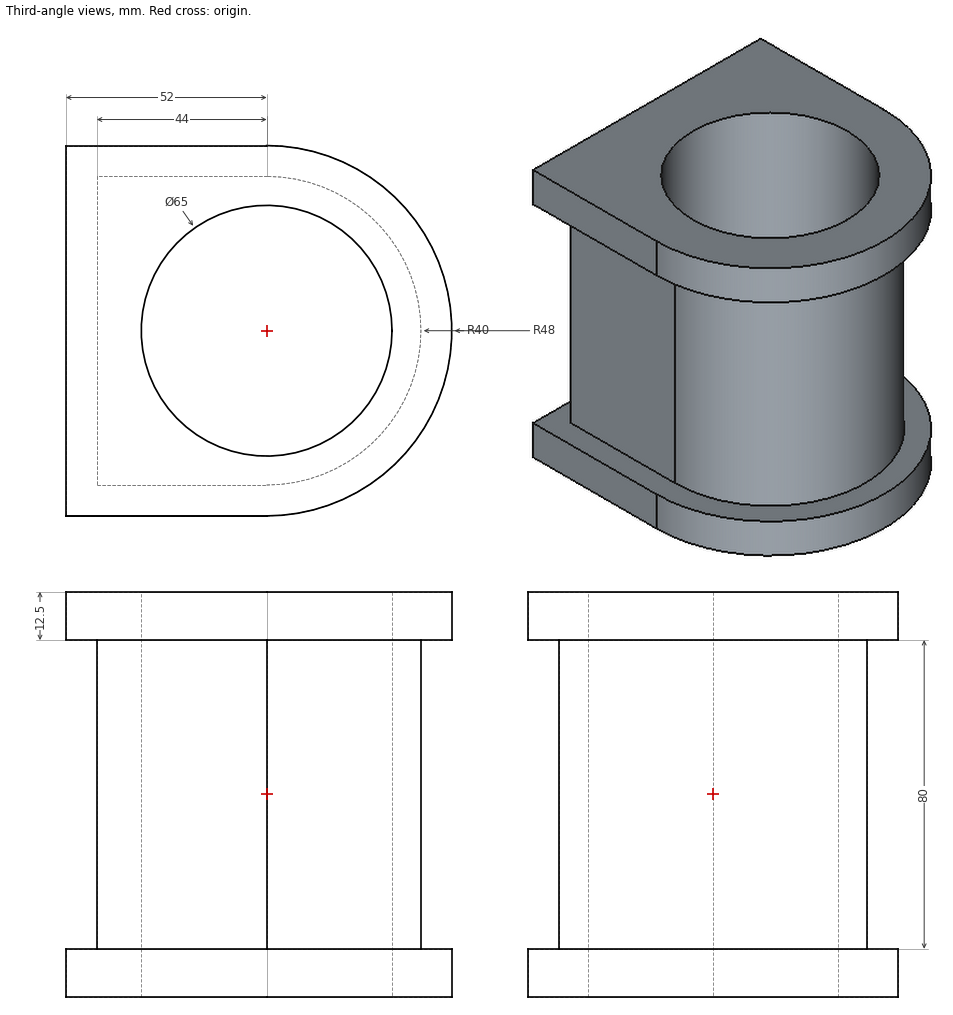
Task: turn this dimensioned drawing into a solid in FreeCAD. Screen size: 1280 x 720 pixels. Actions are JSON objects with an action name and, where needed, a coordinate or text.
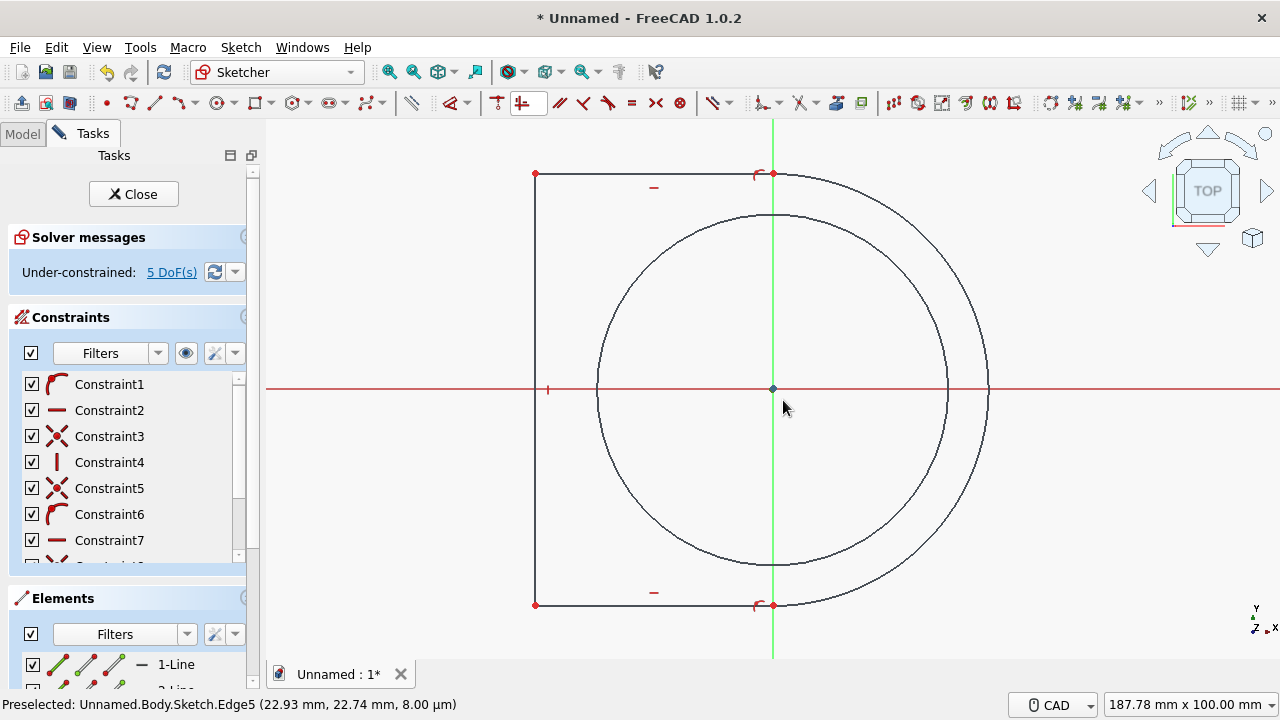
{"action": "left_click", "coordinate": [498, 104]}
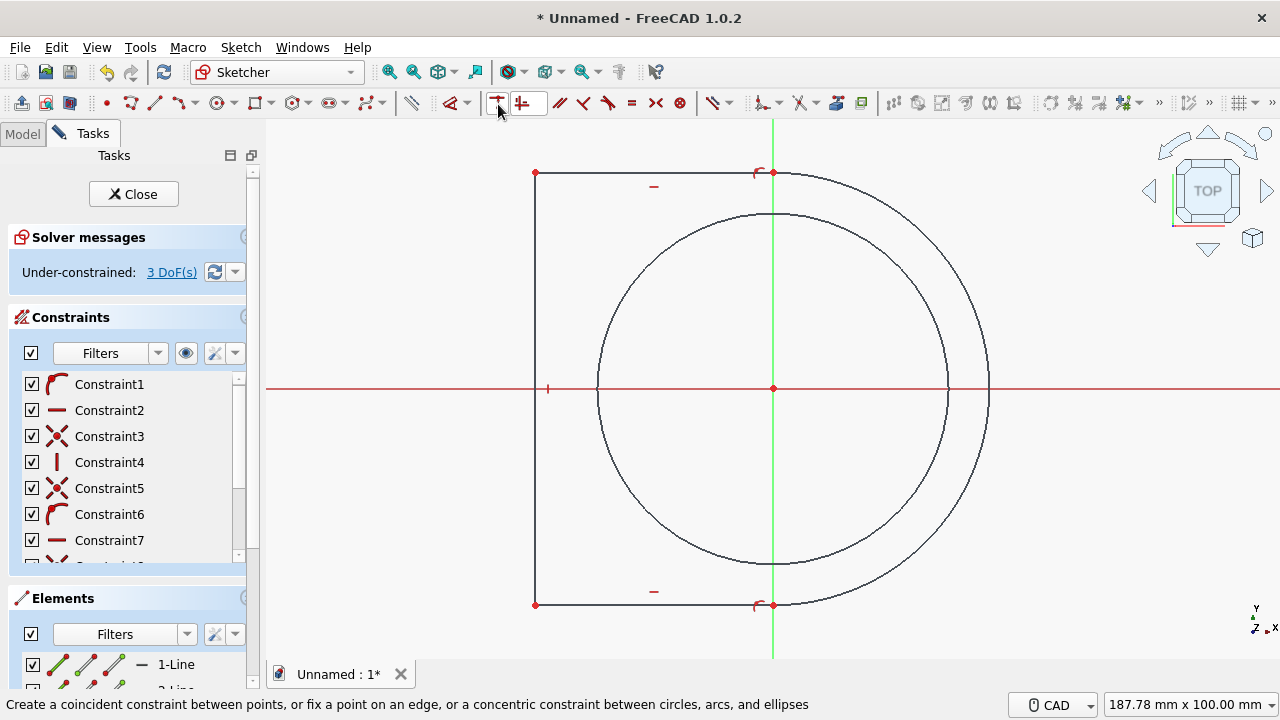
{"action": "left_click", "coordinate": [948, 516]}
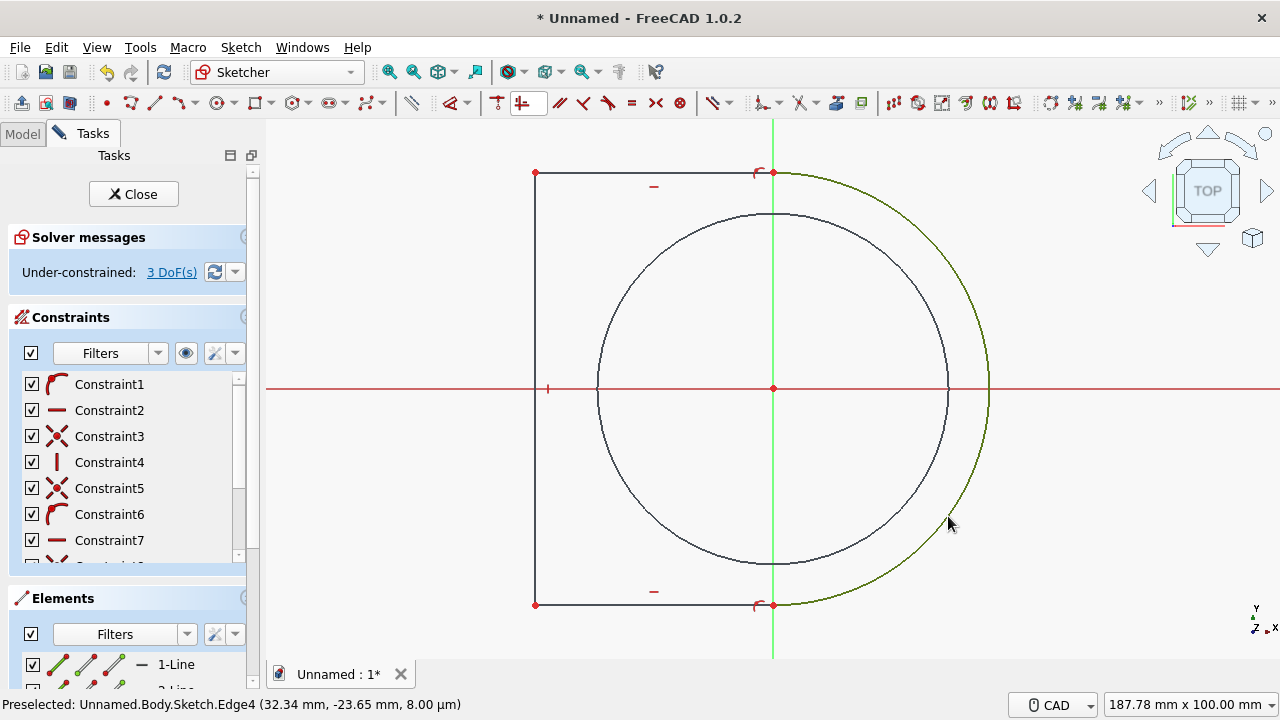
{"action": "key", "text": "k r"}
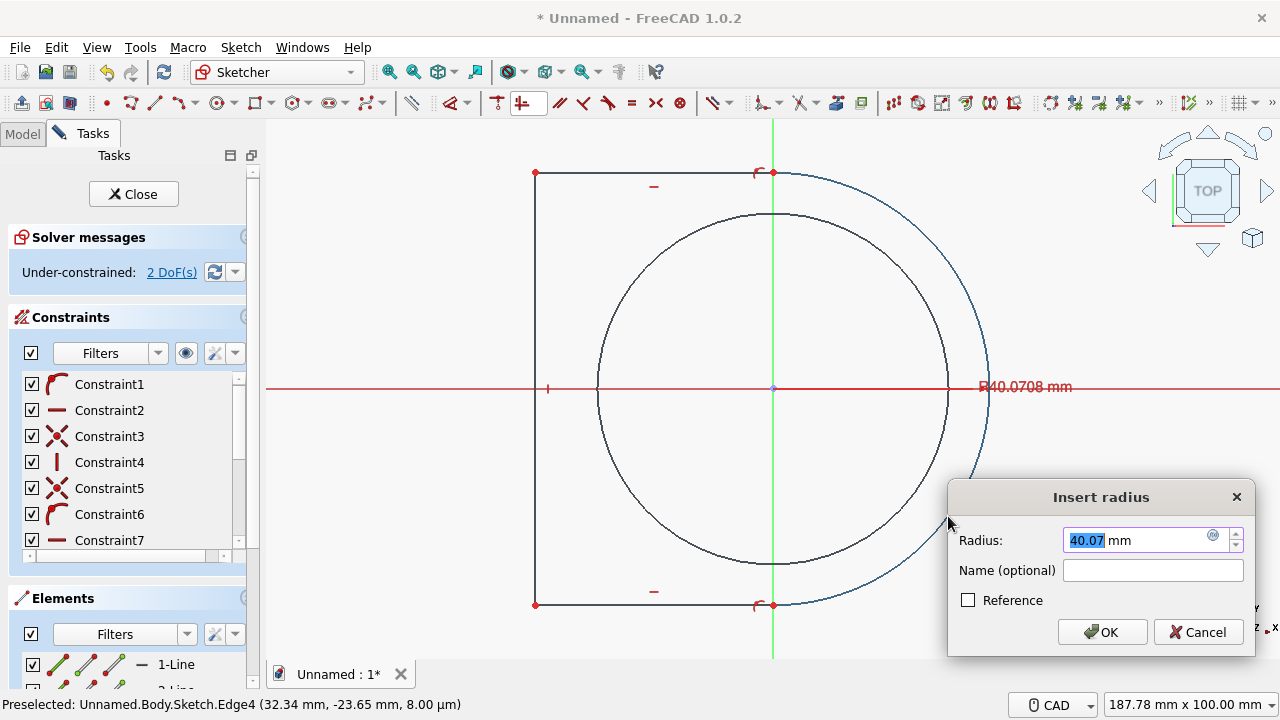
{"action": "type", "text": "40"}
{"action": "key", "text": "Return"}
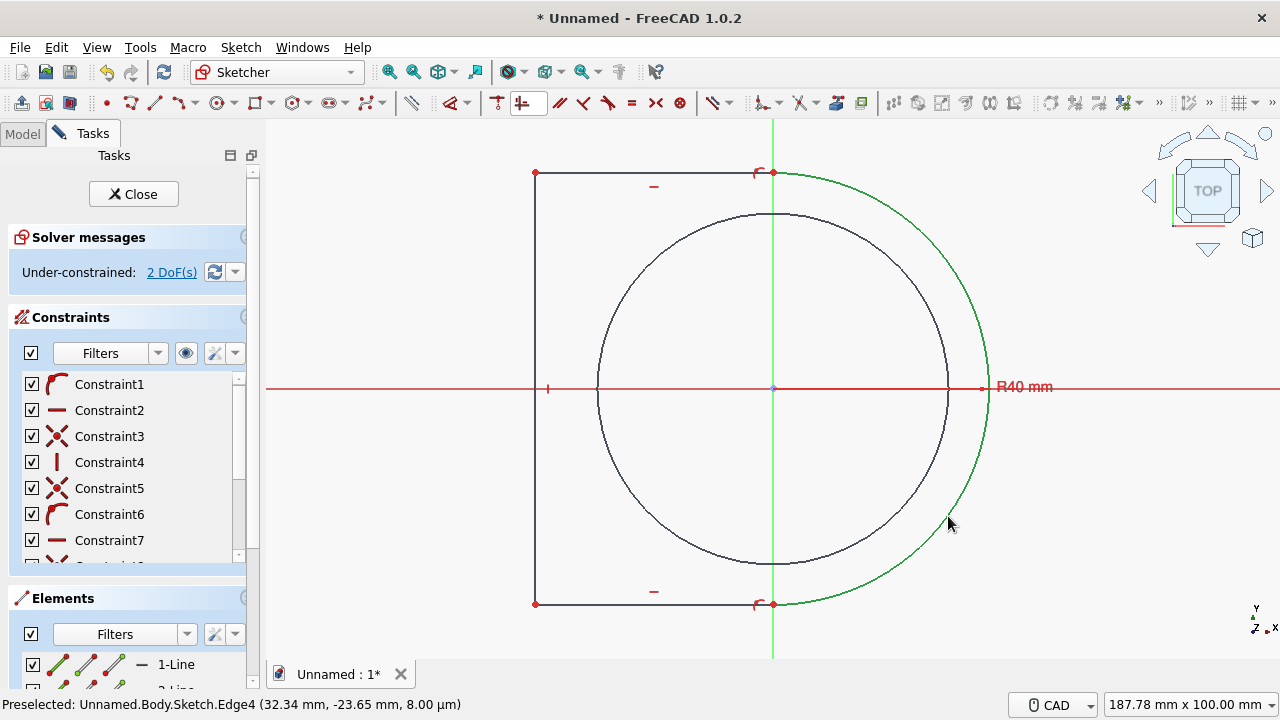
{"action": "left_click", "coordinate": [897, 264]}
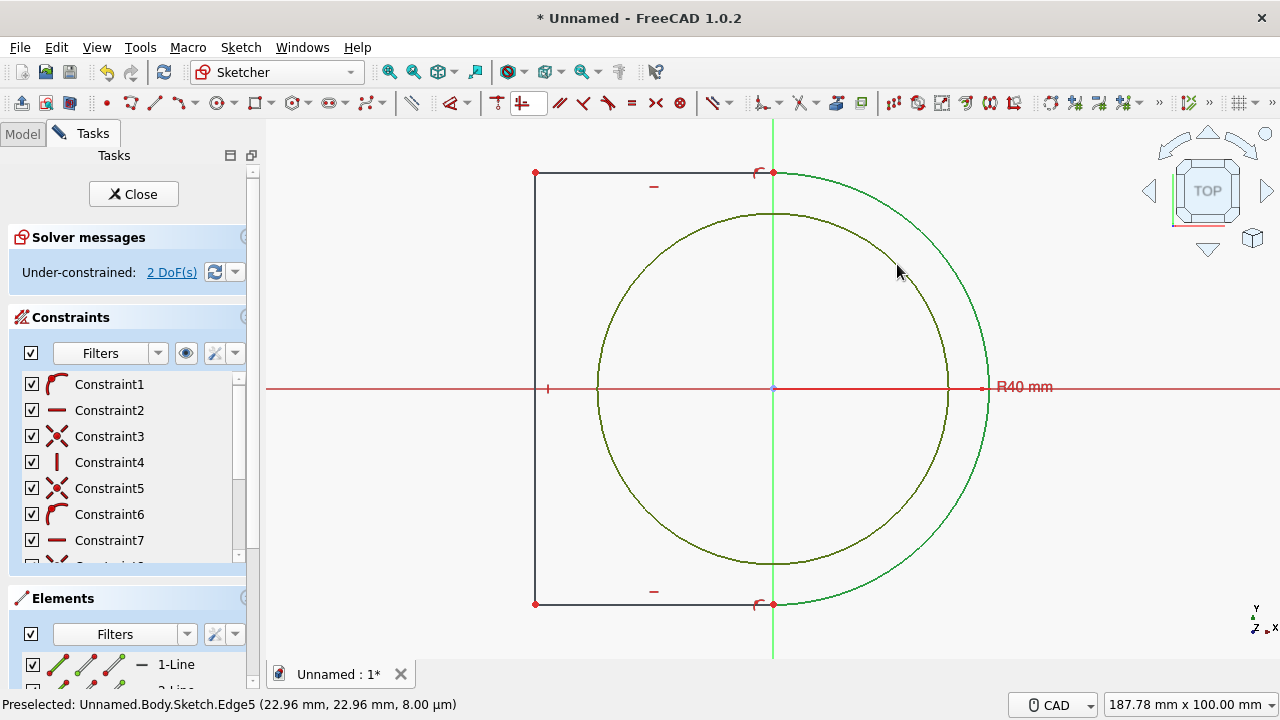
{"action": "key", "text": "k o"}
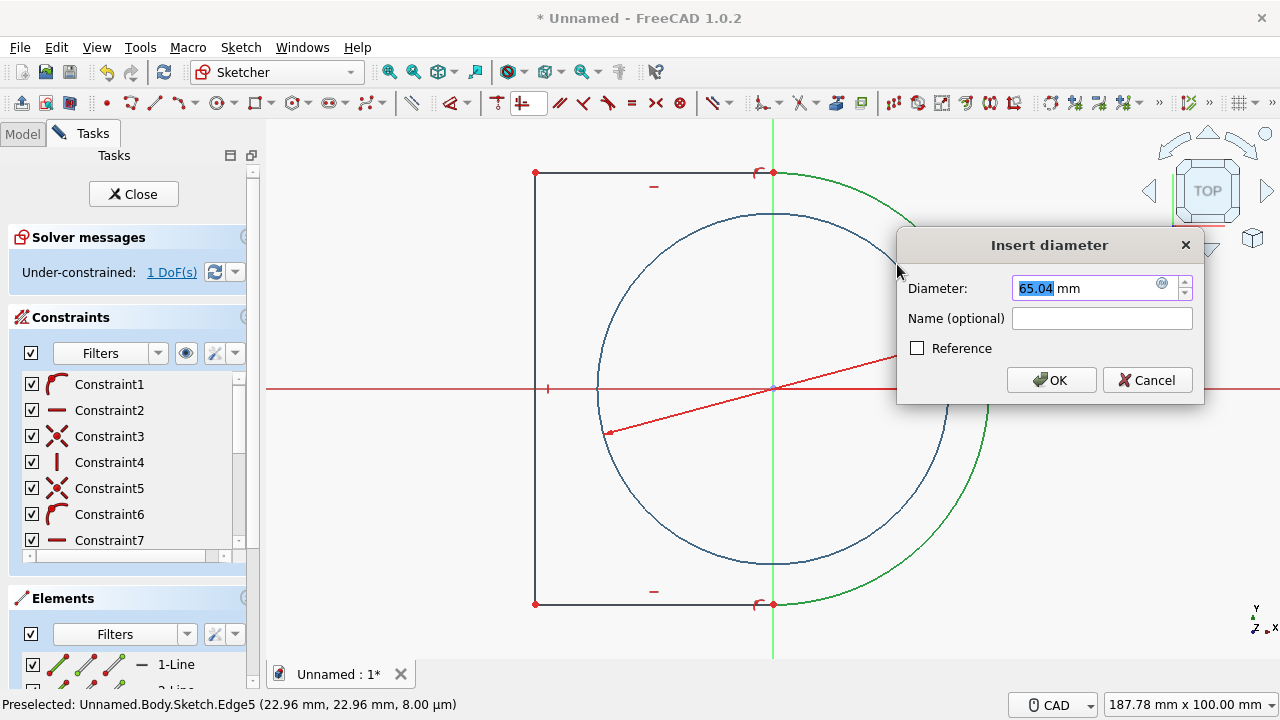
{"action": "type", "text": "65"}
{"action": "key", "text": "Return"}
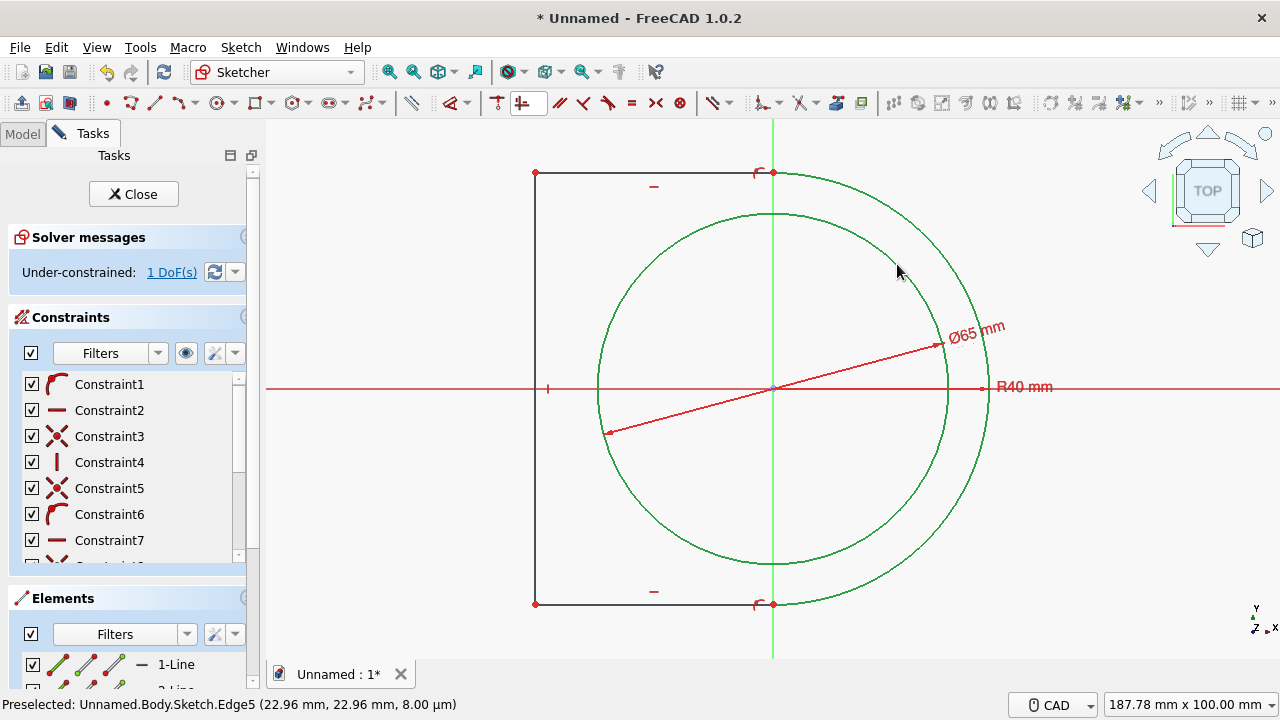
{"action": "left_click", "coordinate": [702, 173]}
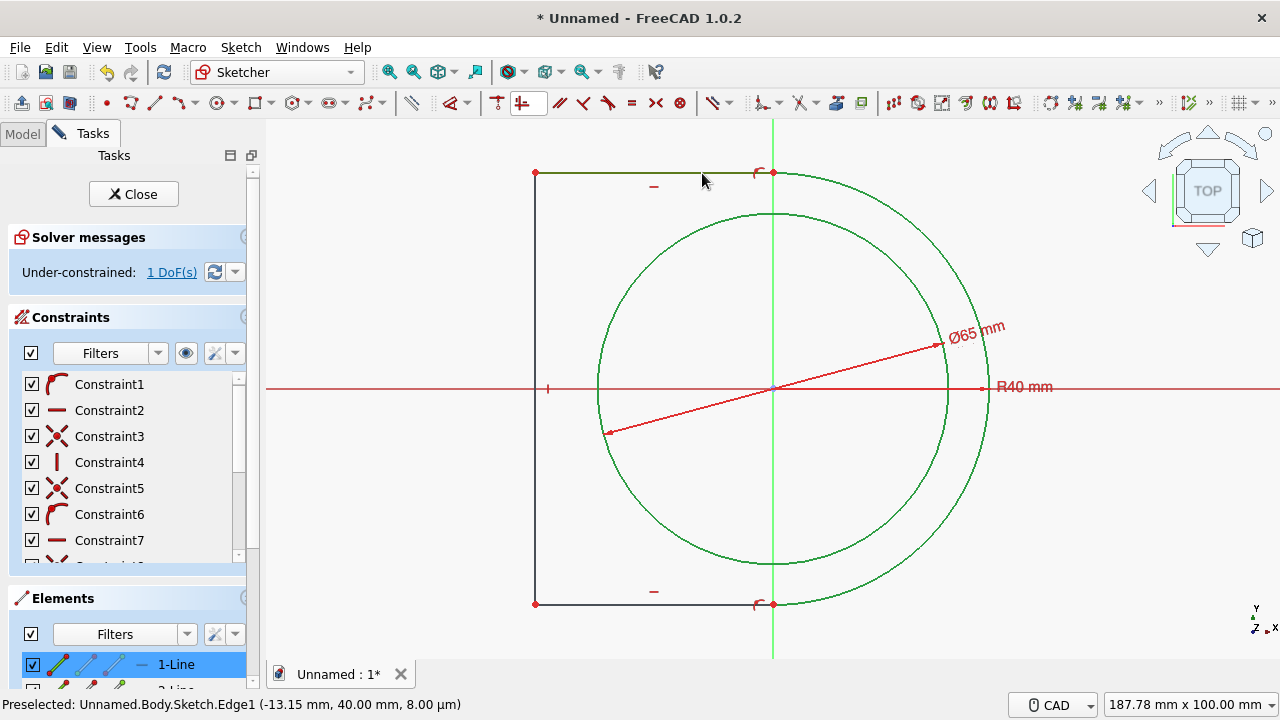
{"action": "key", "text": "l"}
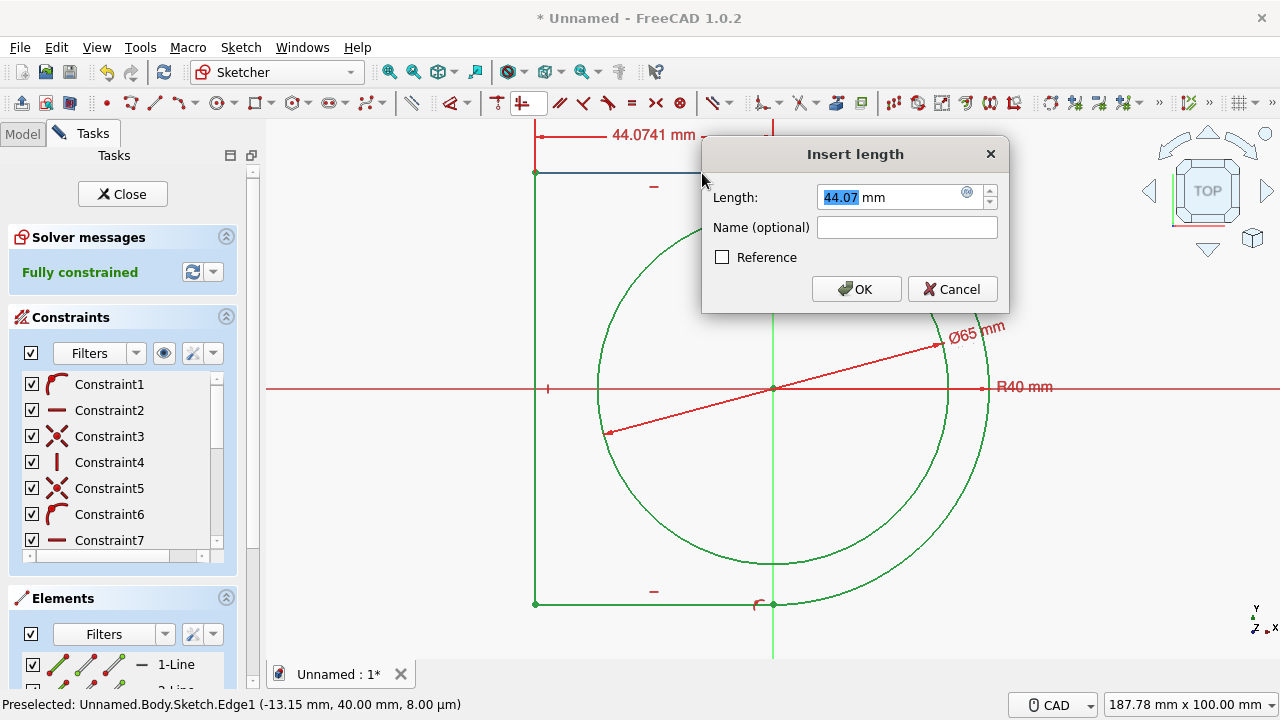
{"action": "type", "text": "44"}
{"action": "key", "text": "Return"}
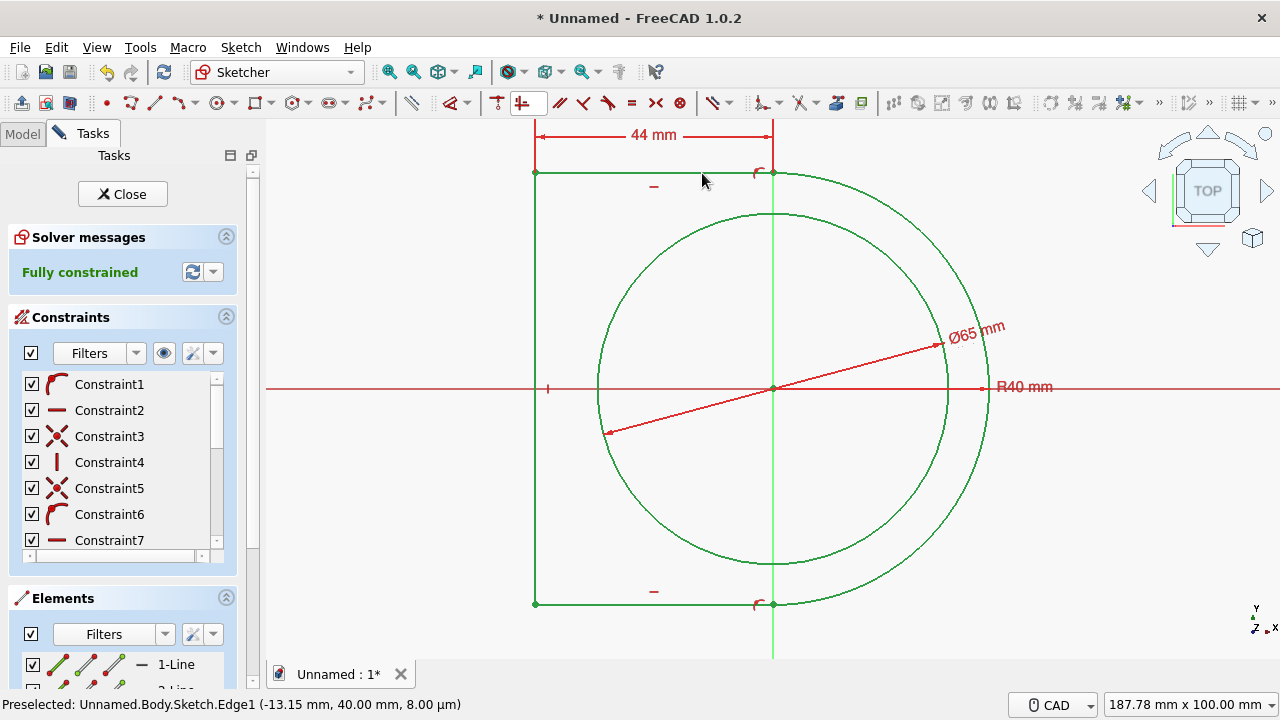
{"action": "left_click", "coordinate": [123, 194]}